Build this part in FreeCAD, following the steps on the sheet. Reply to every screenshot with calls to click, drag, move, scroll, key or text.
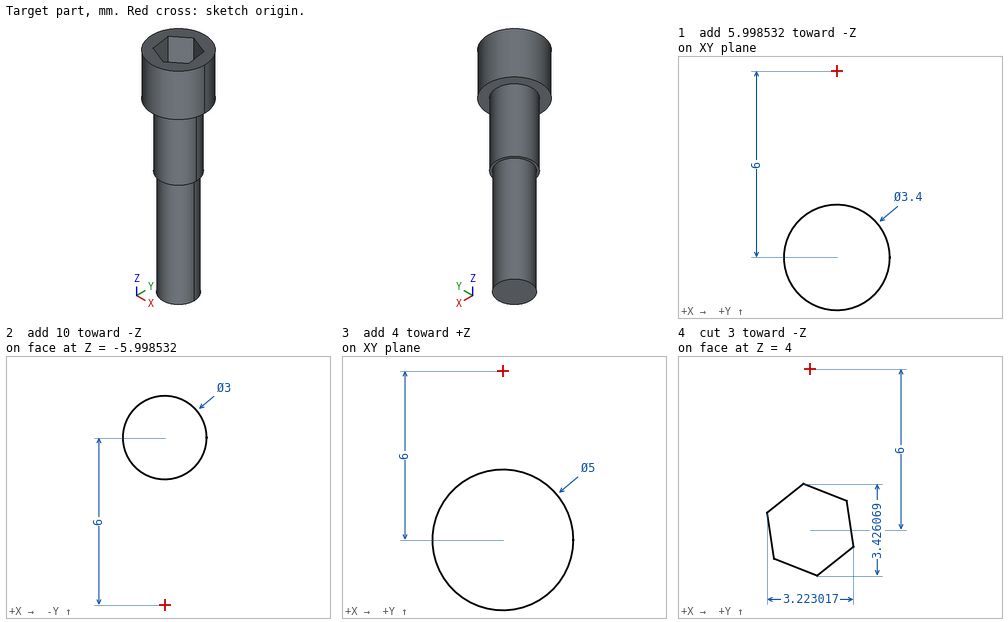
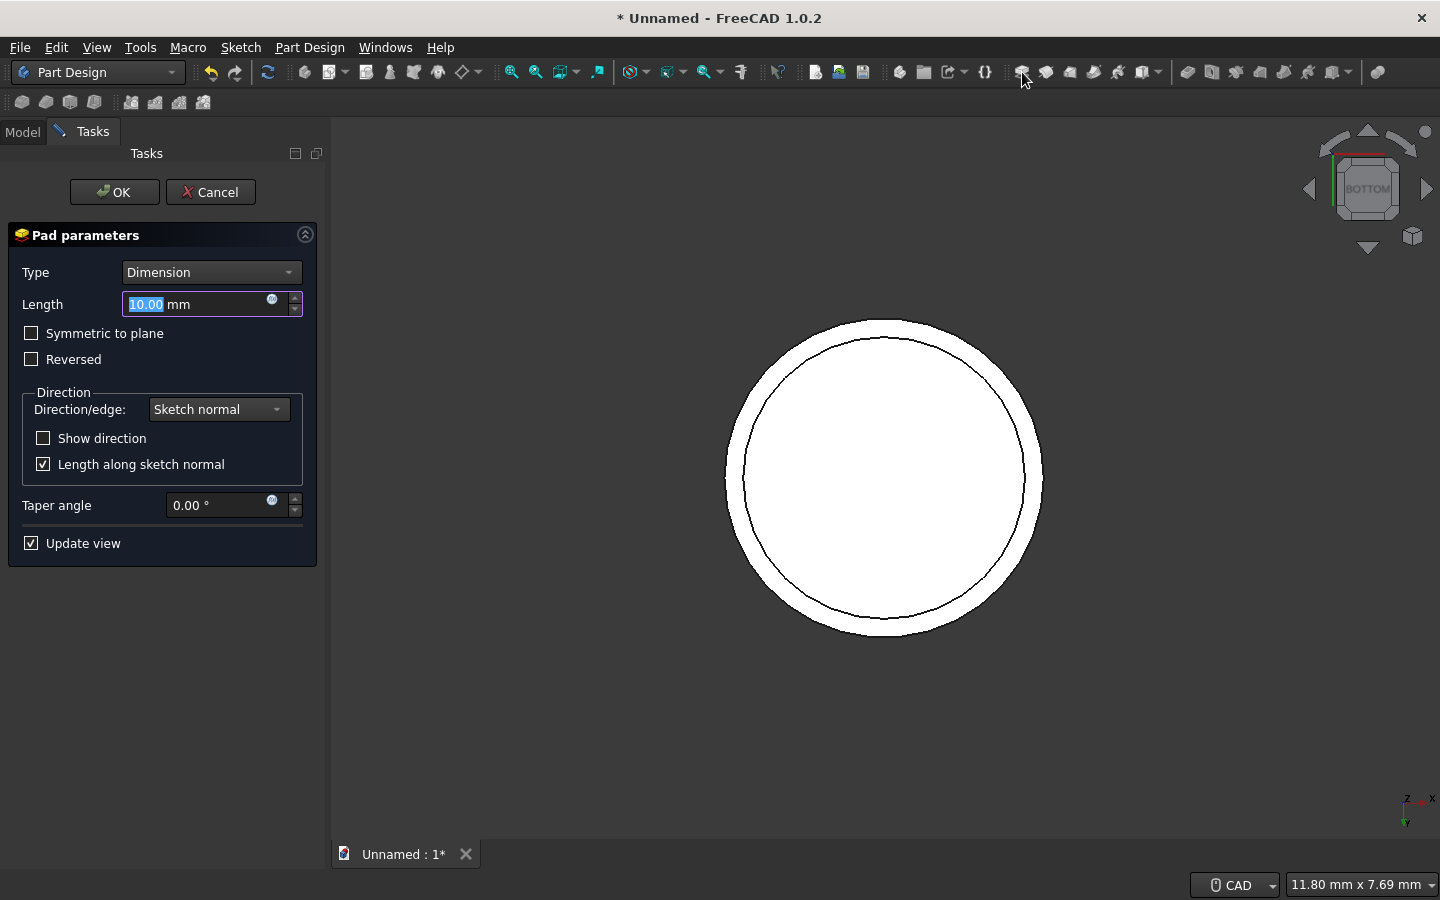
text(10)
key(Tab)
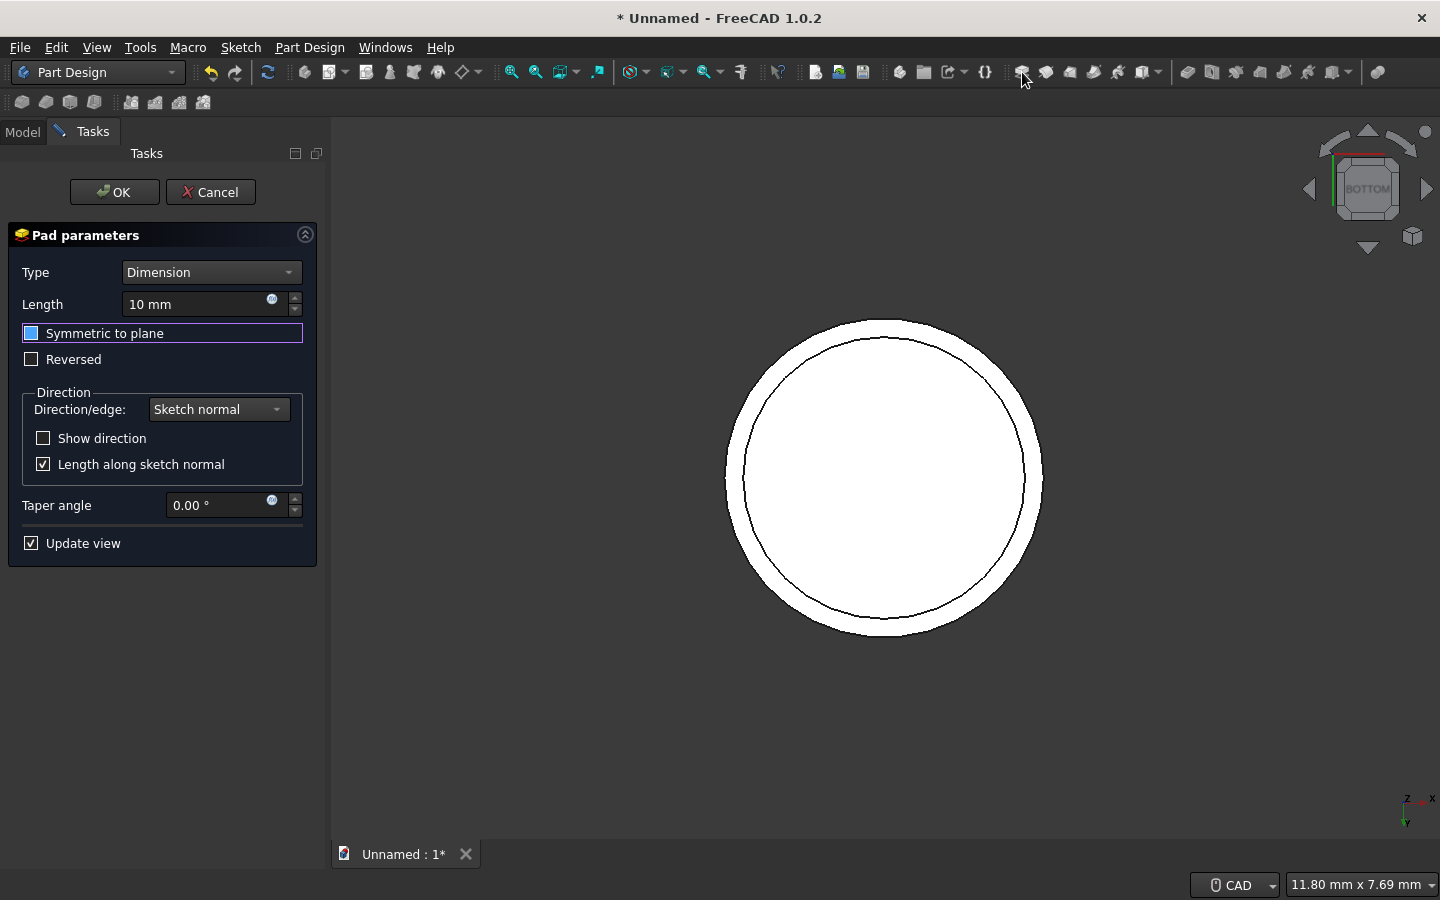
click(115, 192)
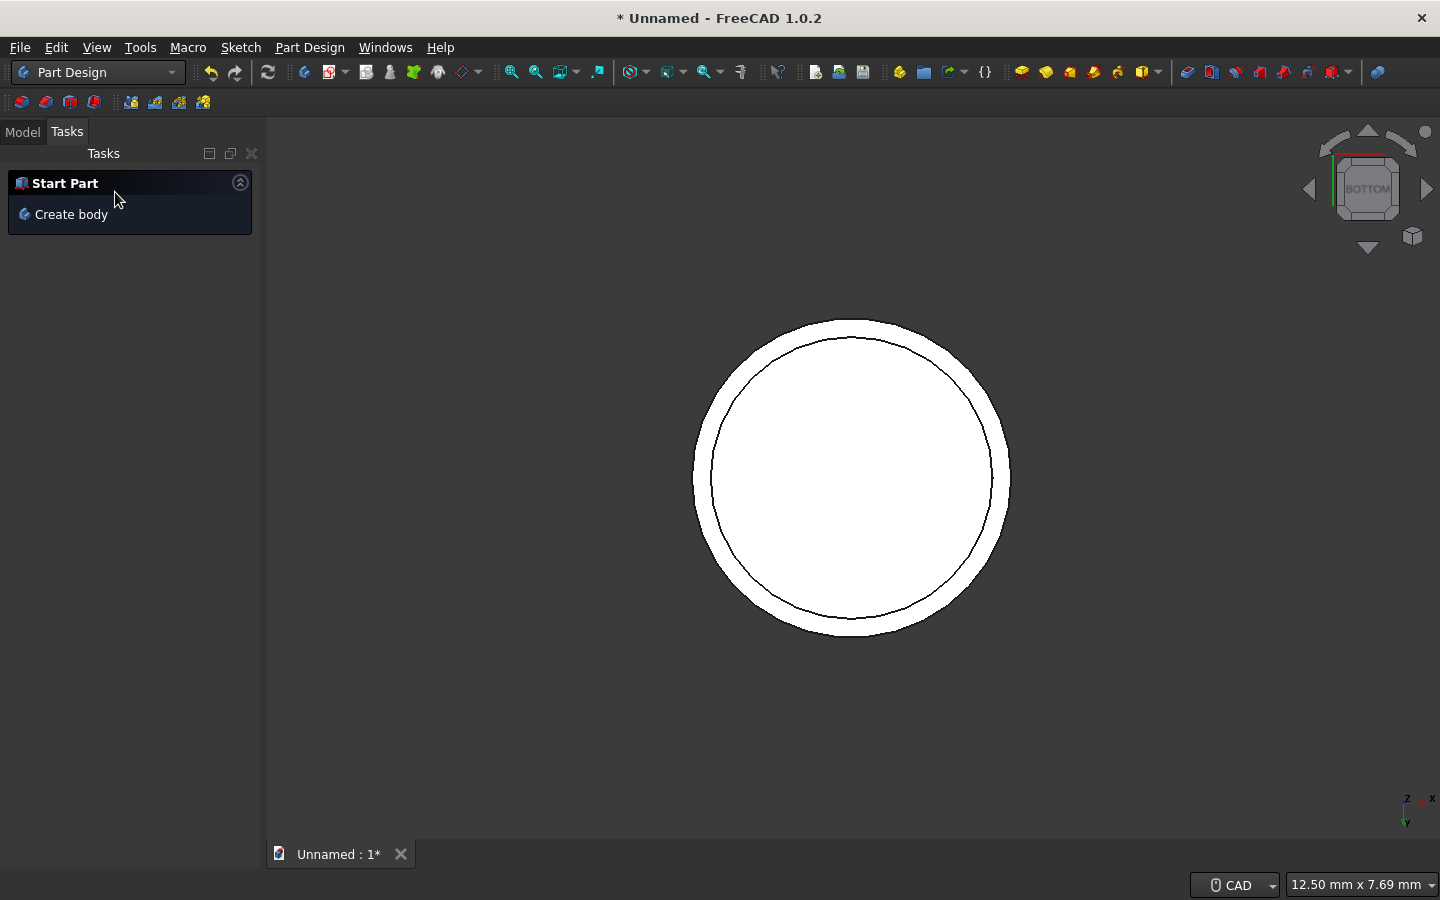
key(v)
key(f)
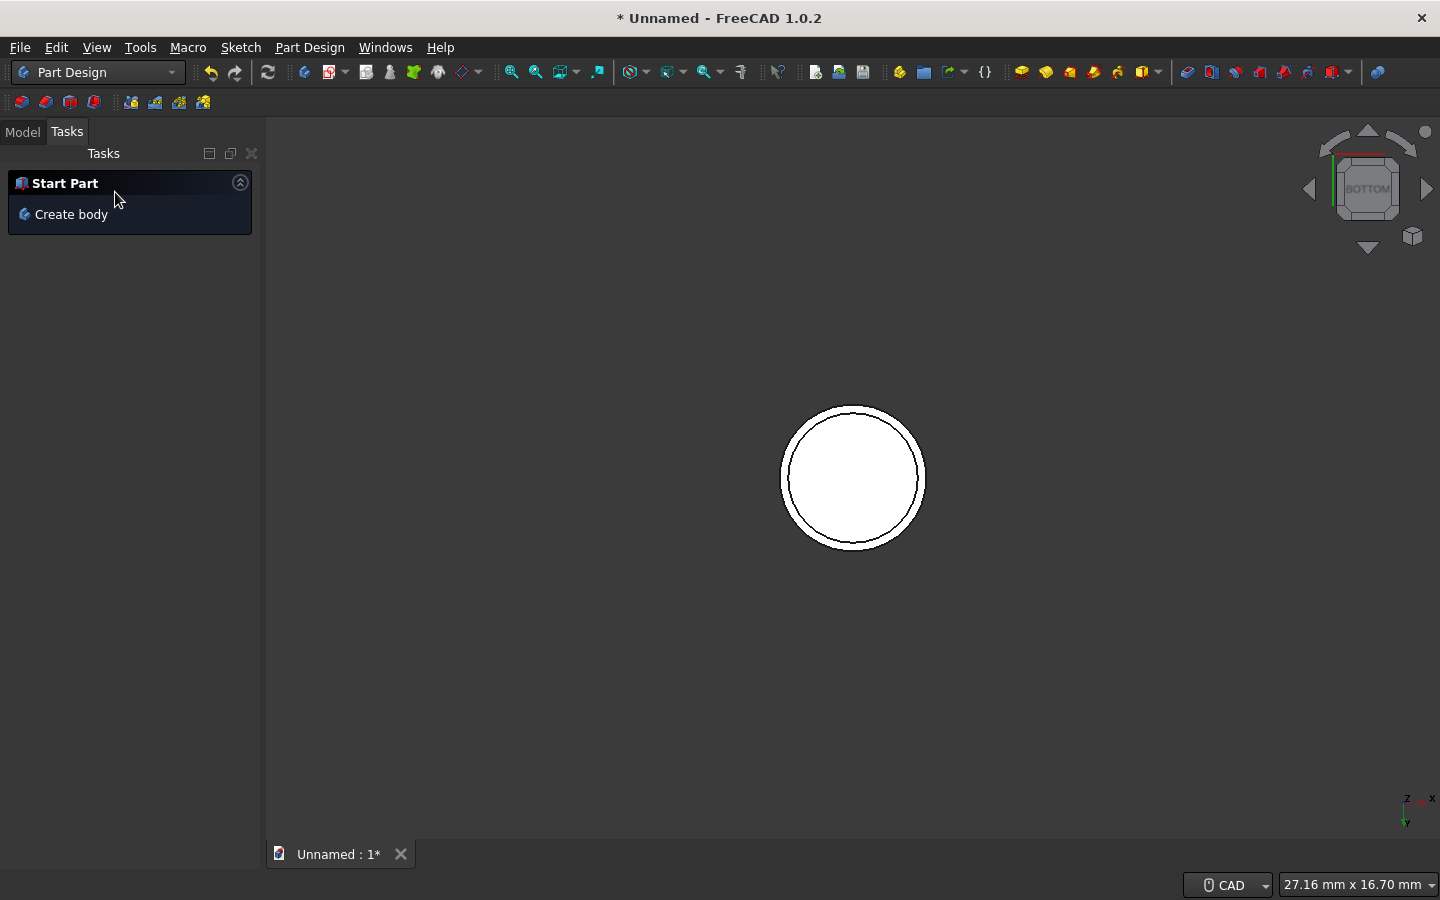
click(330, 72)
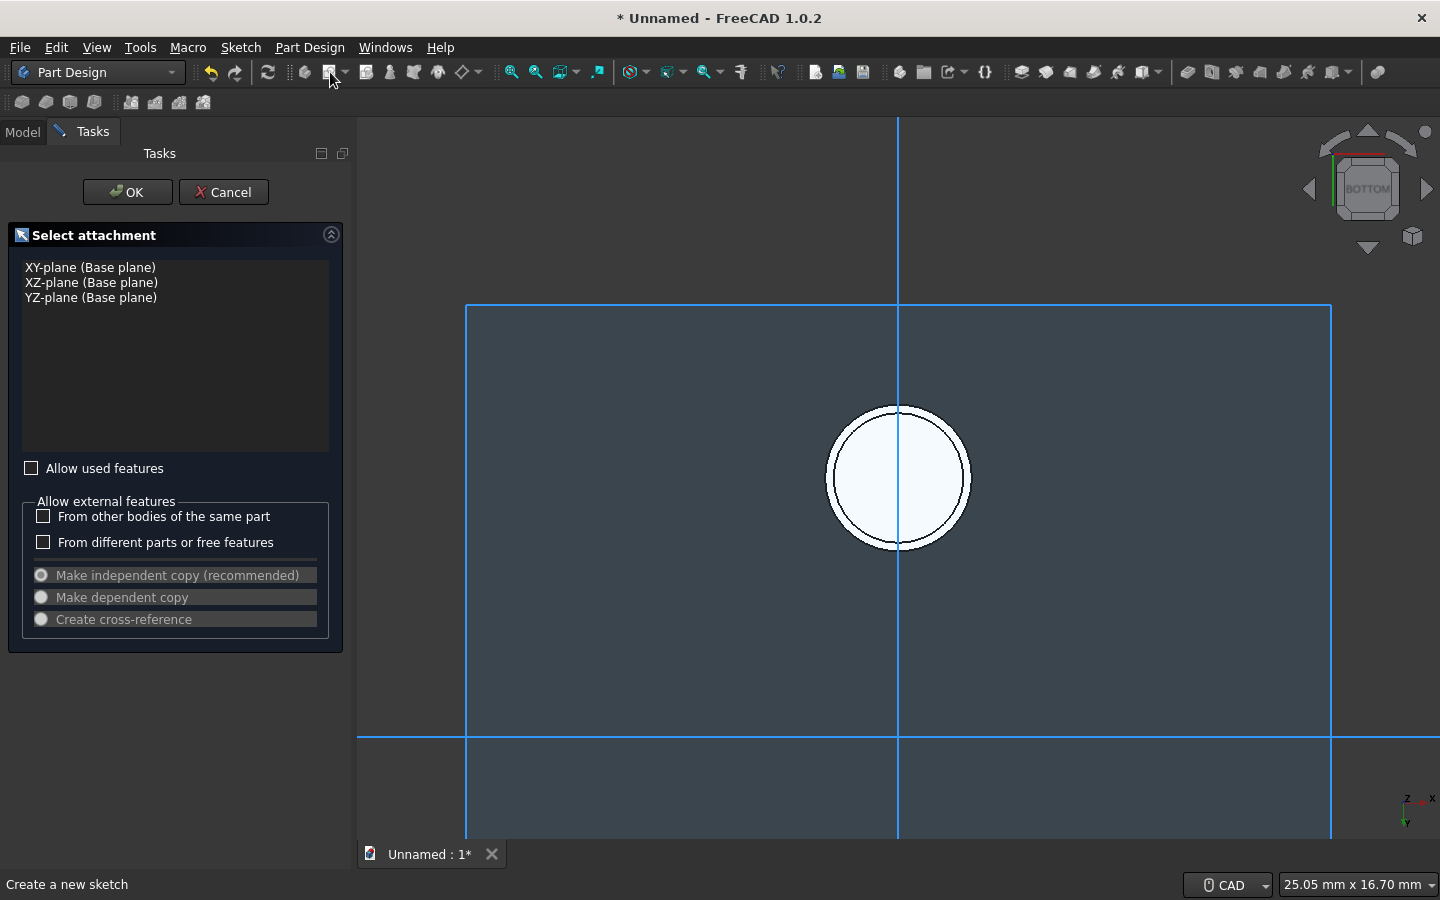
click(82, 268)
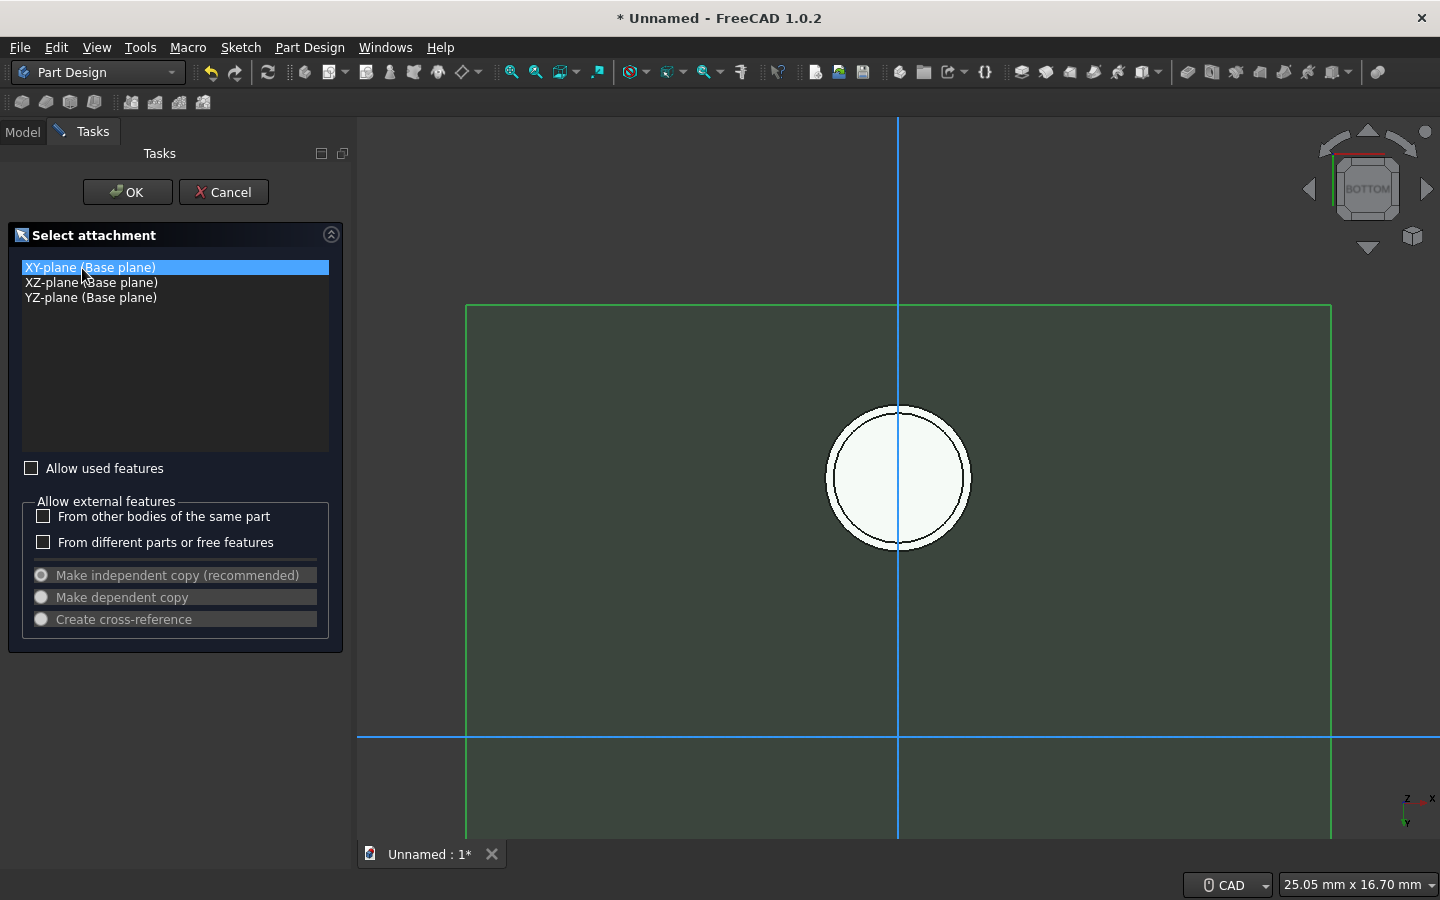
click(128, 192)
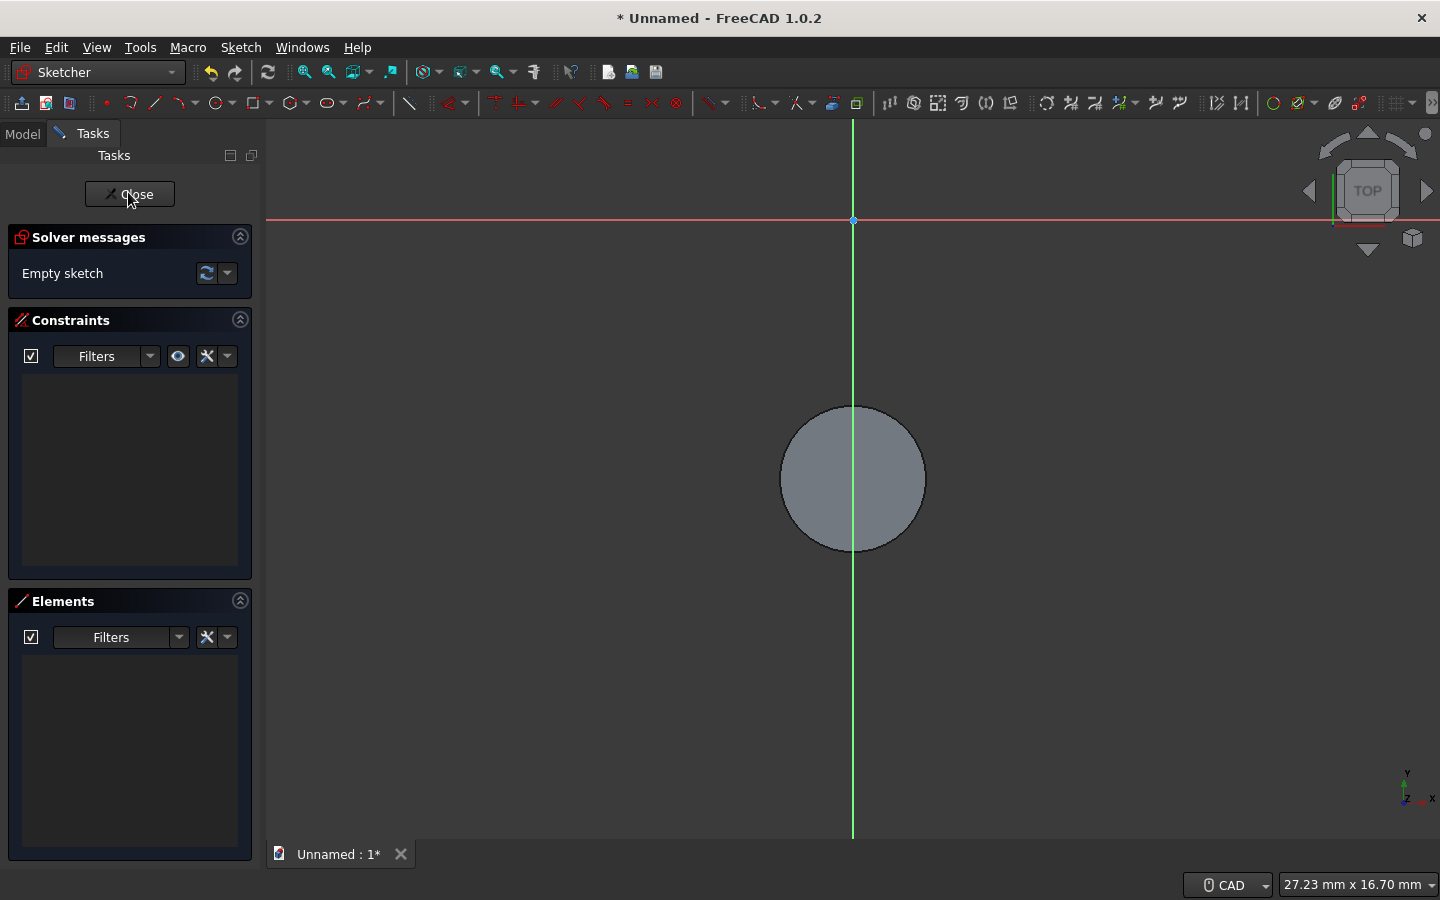
click(216, 104)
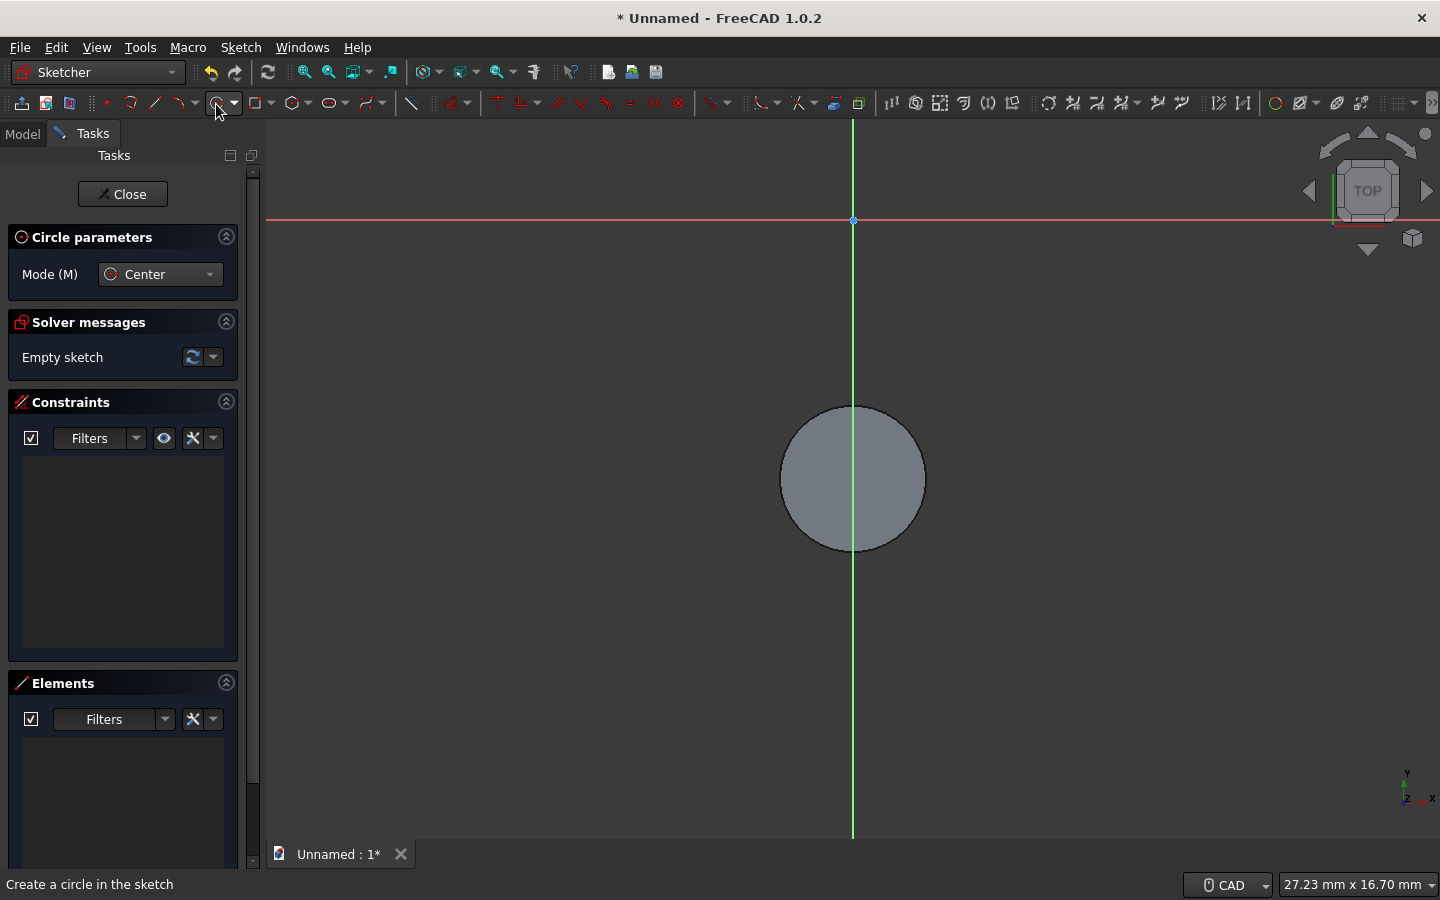
click(853, 479)
click(929, 403)
key(Escape)